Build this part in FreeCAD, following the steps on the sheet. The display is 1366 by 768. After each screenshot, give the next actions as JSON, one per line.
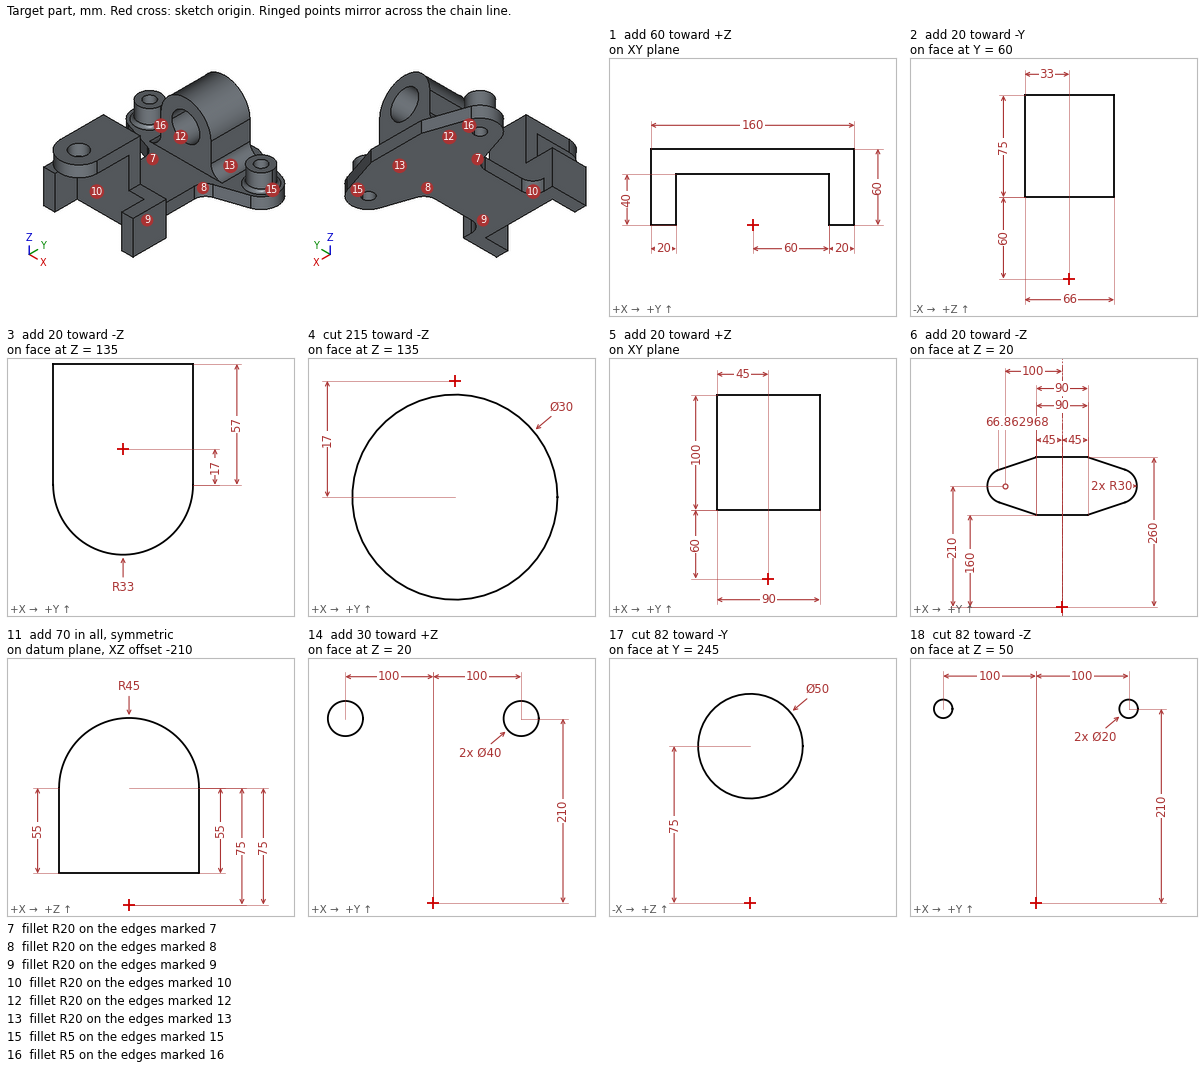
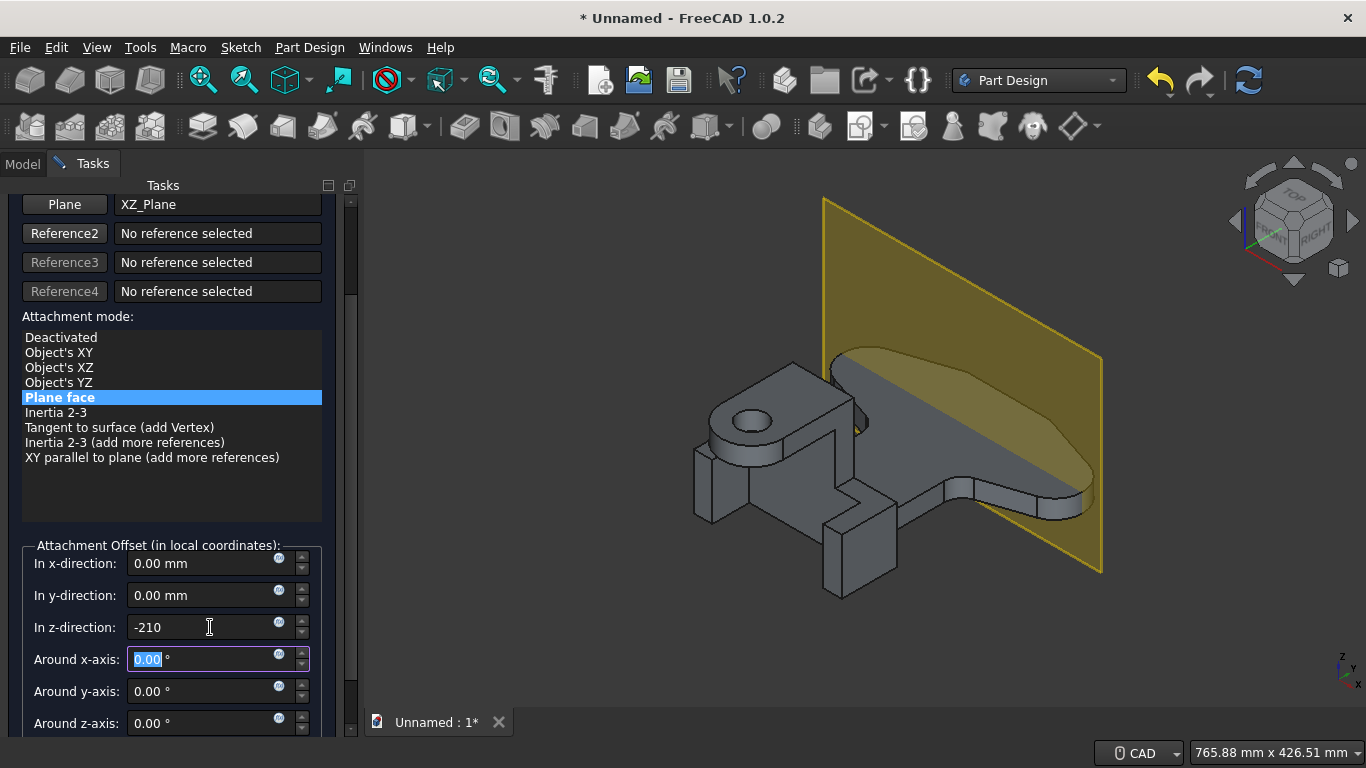
{"action": "scroll", "coordinate": [351, 466], "scroll_direction": "up", "scroll_amount": 3}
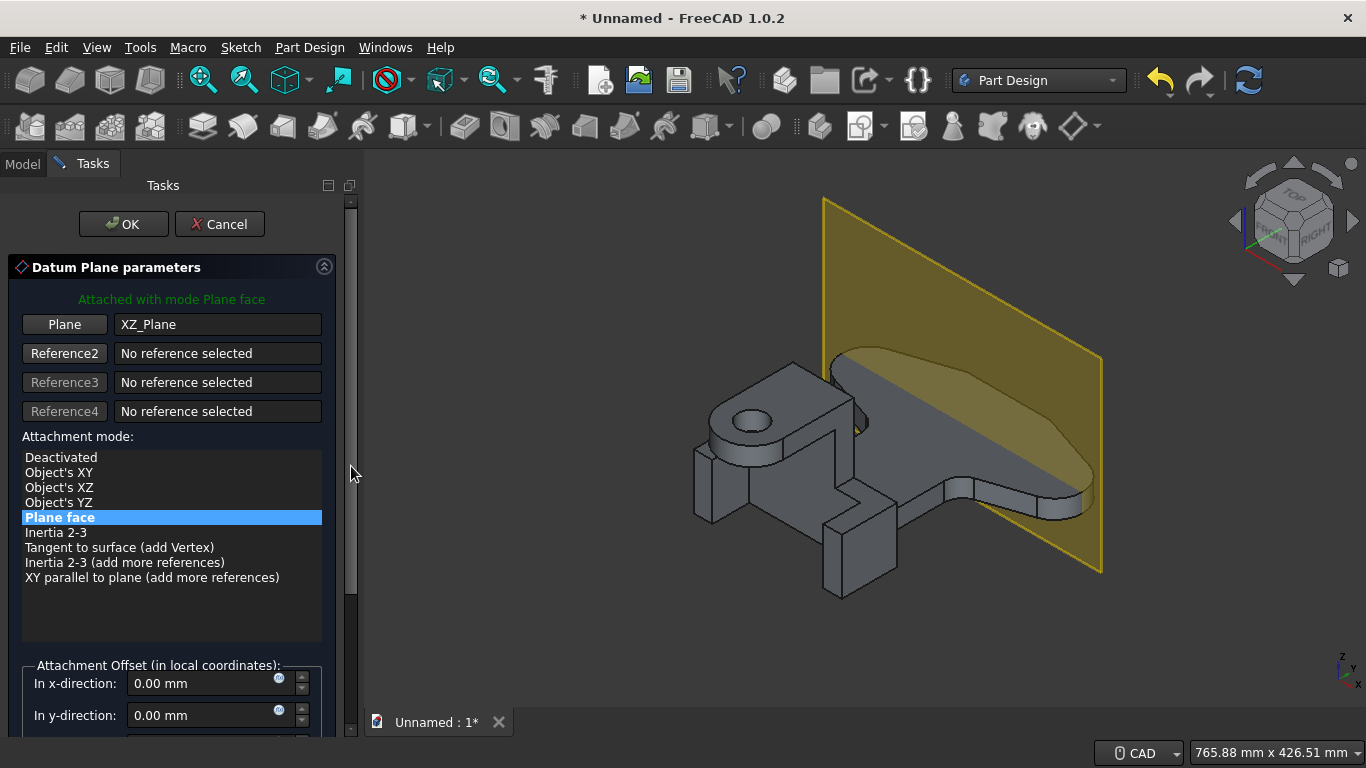
{"action": "left_click", "coordinate": [124, 224]}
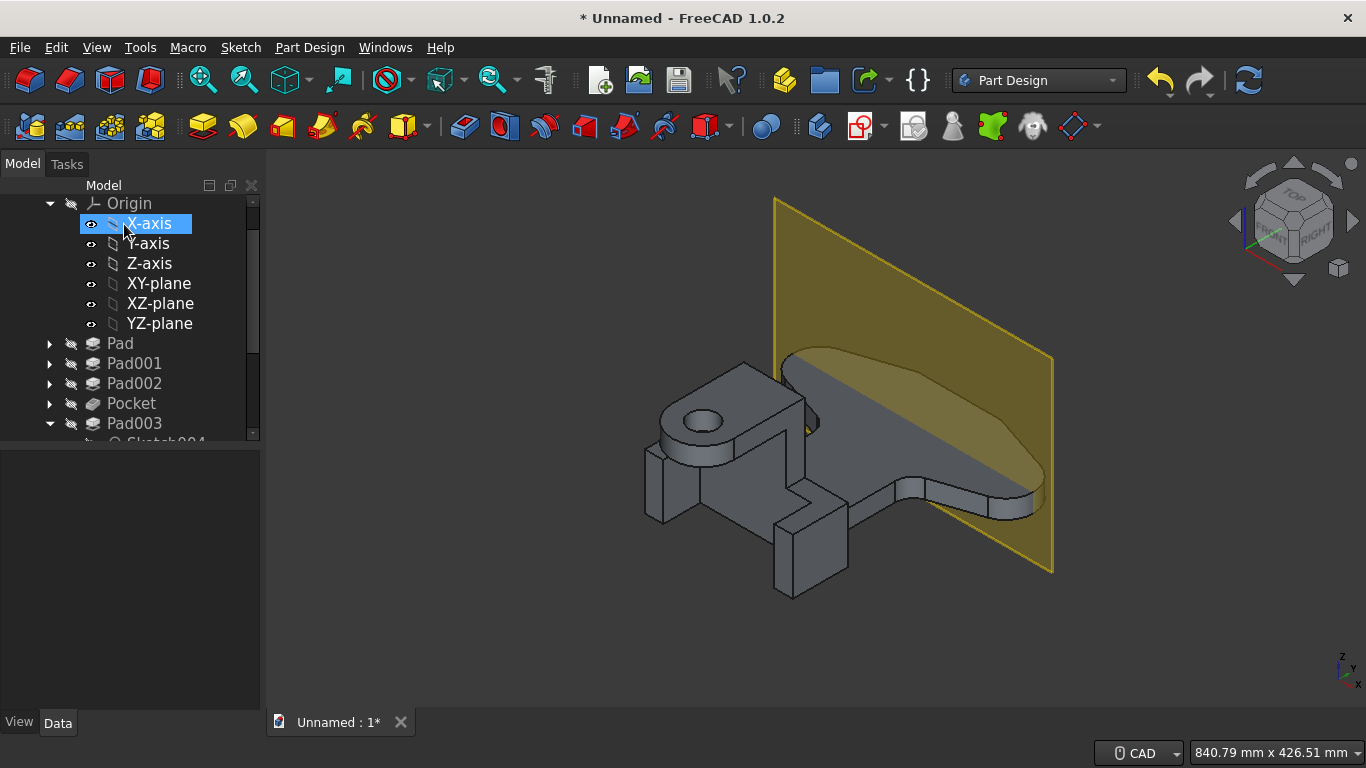
{"action": "scroll", "coordinate": [140, 319], "scroll_direction": "down", "scroll_amount": 3}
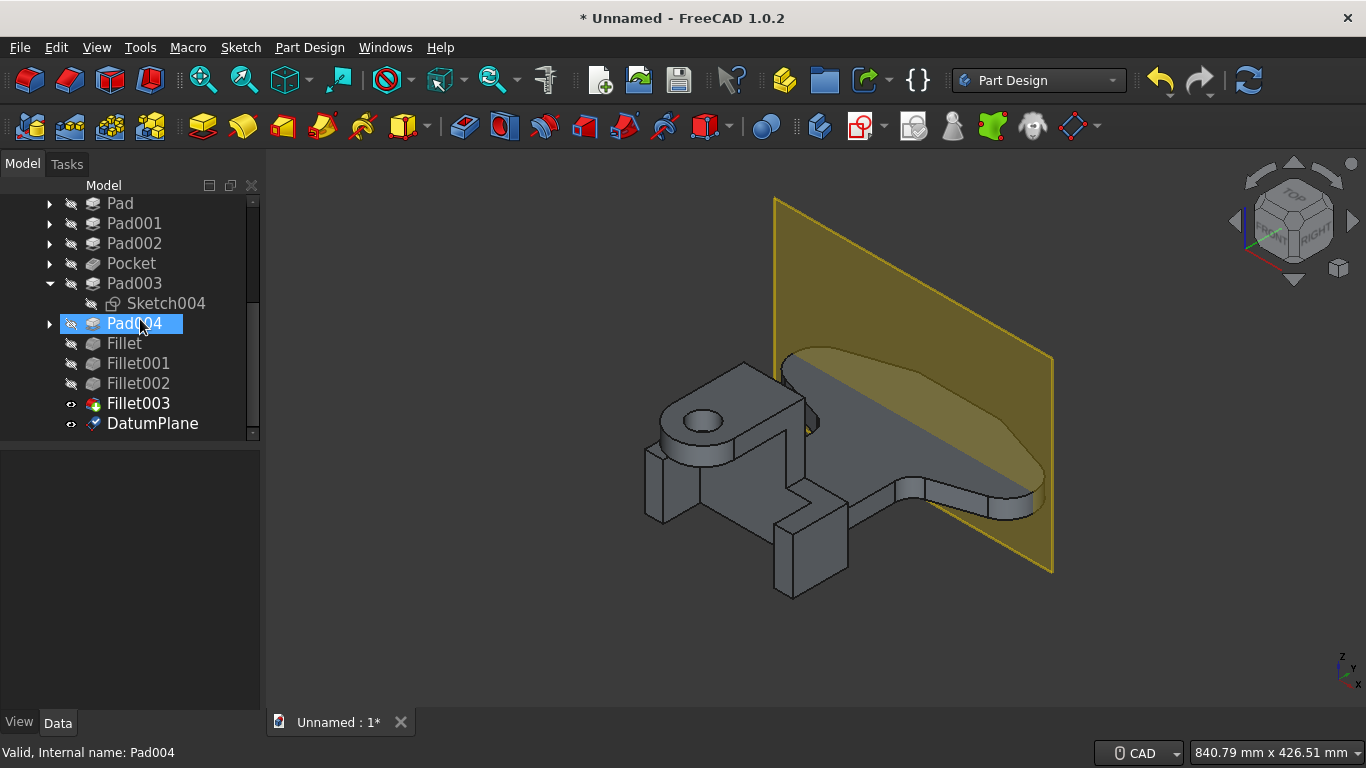
{"action": "left_click", "coordinate": [116, 424]}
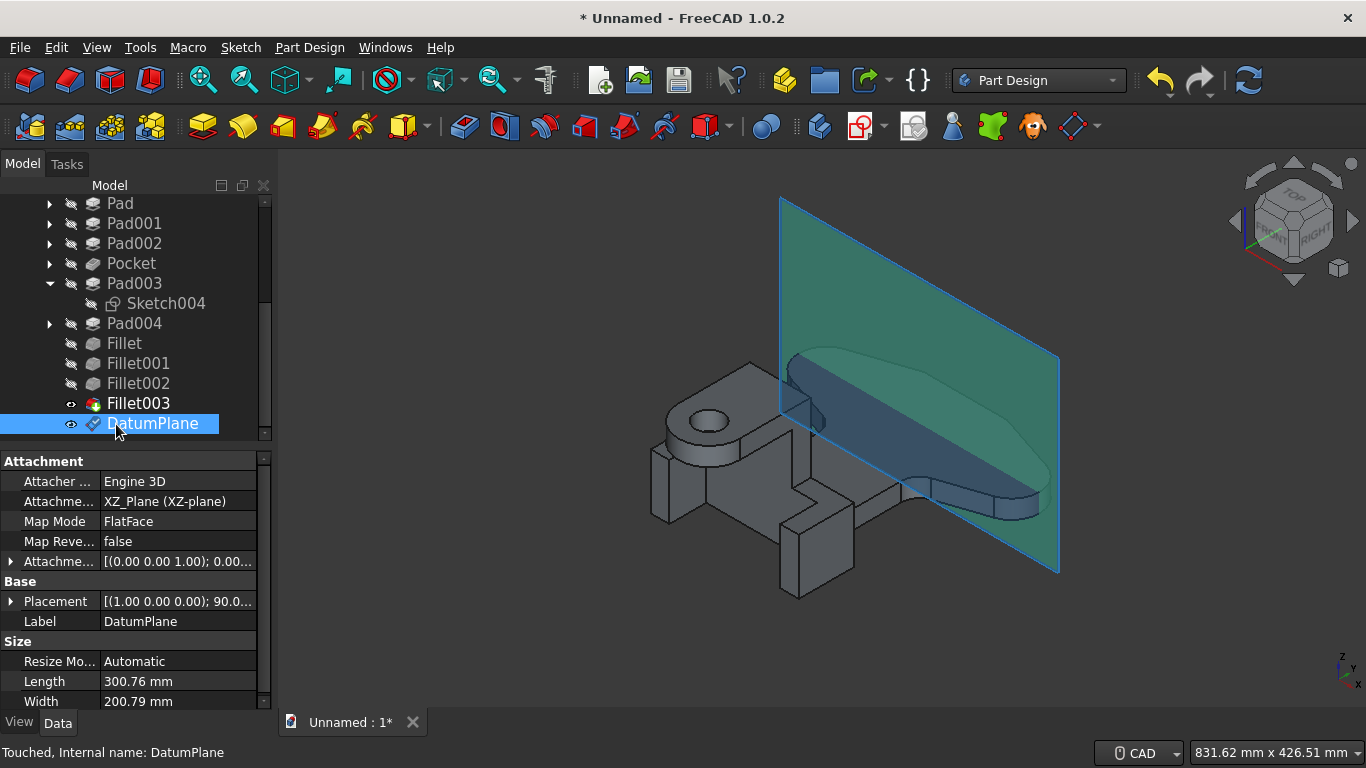
{"action": "left_click", "coordinate": [860, 126]}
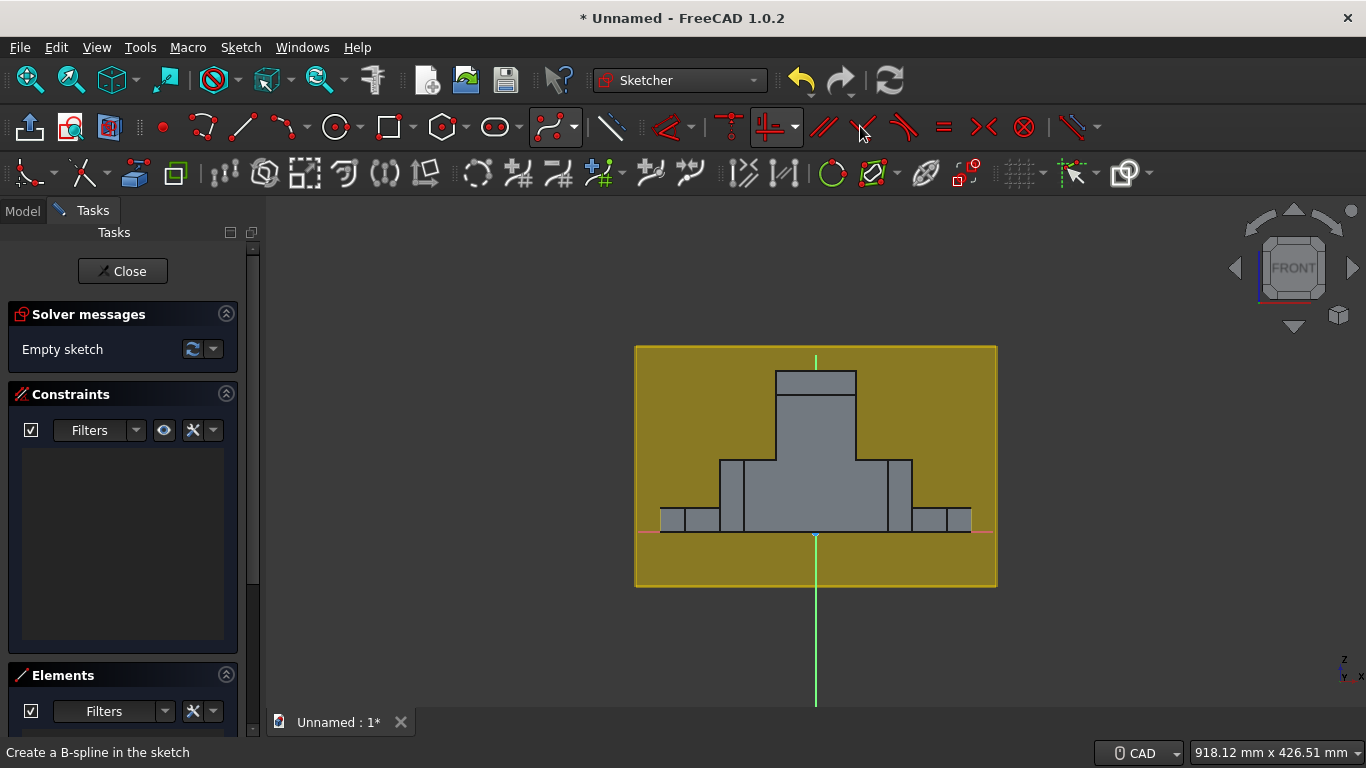
{"action": "key", "text": "q s"}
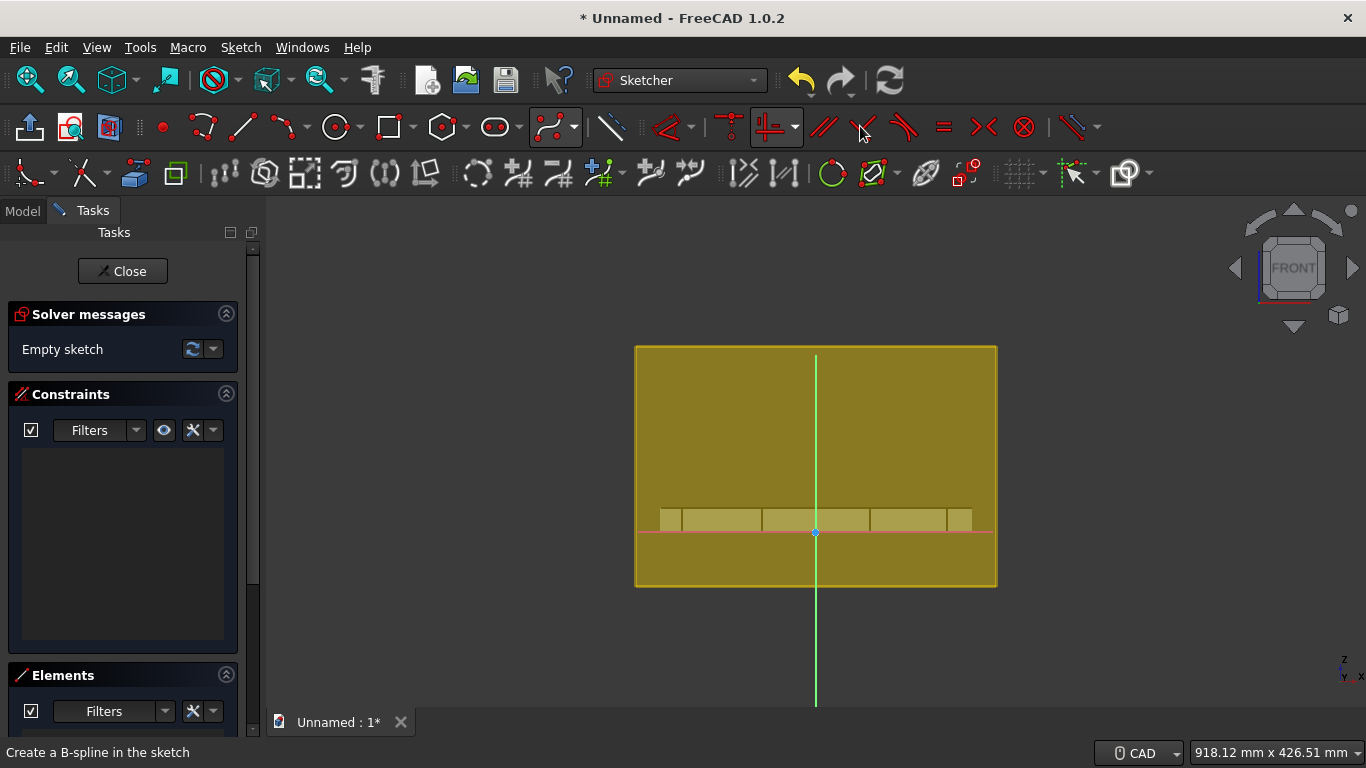
{"action": "scroll", "coordinate": [872, 468], "scroll_direction": "up", "scroll_amount": 4}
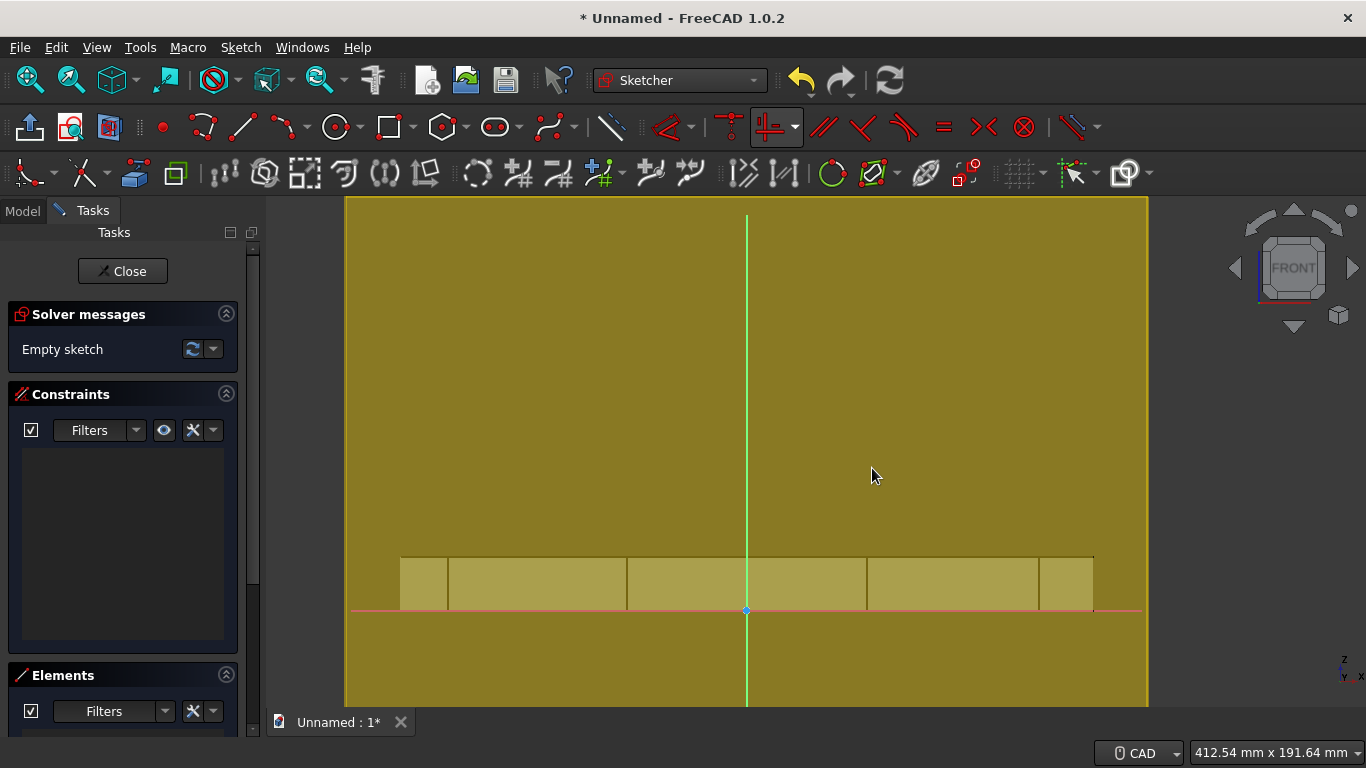
{"action": "key", "text": "g m"}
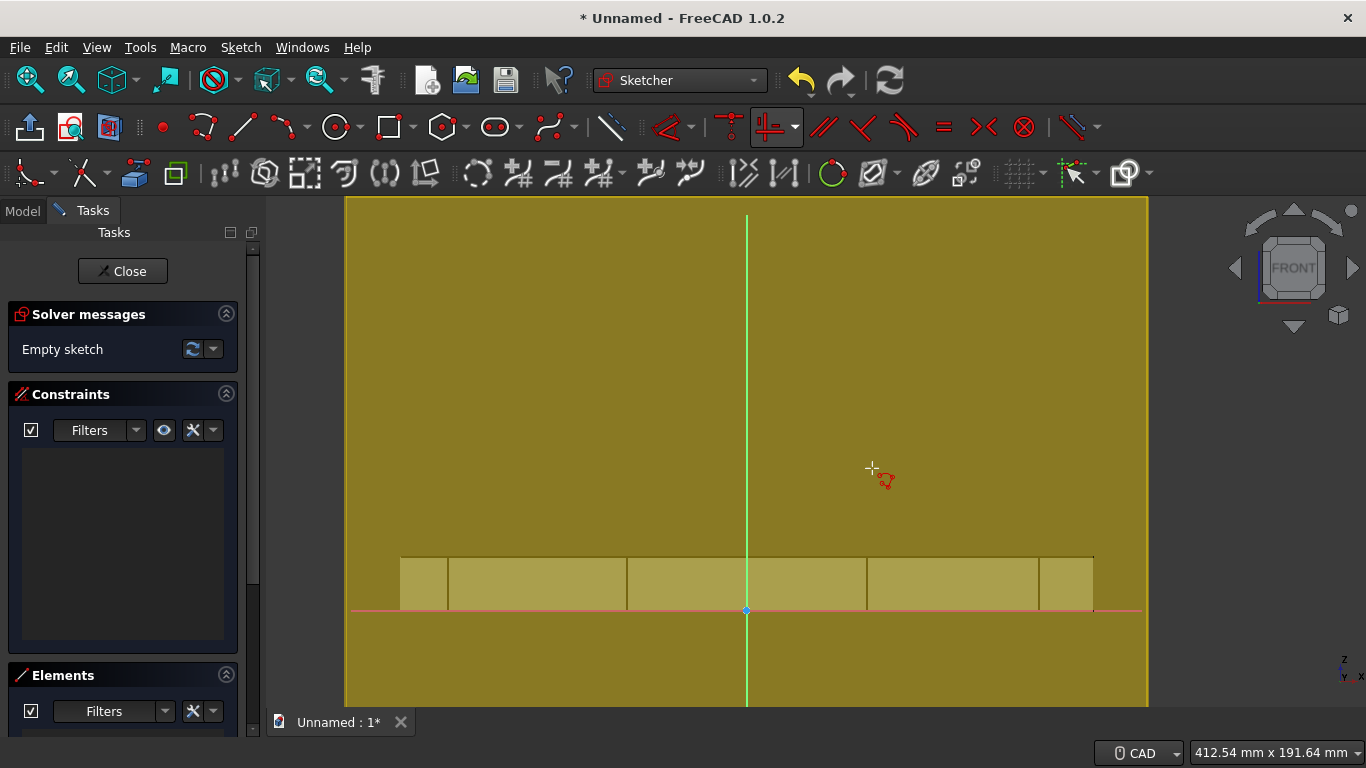
{"action": "left_click", "coordinate": [867, 411]}
{"action": "left_click", "coordinate": [867, 557]}
{"action": "left_click", "coordinate": [627, 557]}
{"action": "left_click", "coordinate": [627, 411]}
{"action": "right_click", "coordinate": [627, 411]}